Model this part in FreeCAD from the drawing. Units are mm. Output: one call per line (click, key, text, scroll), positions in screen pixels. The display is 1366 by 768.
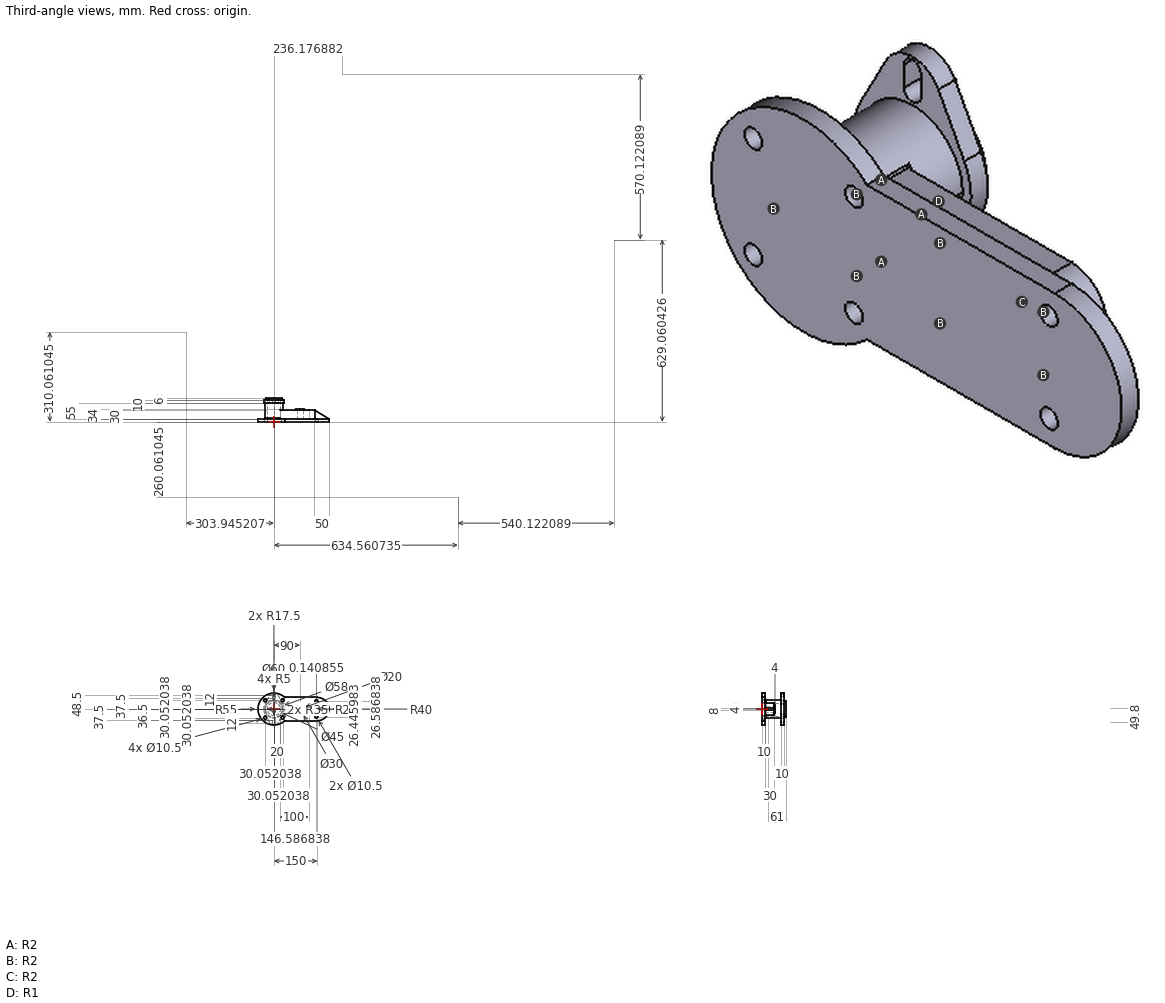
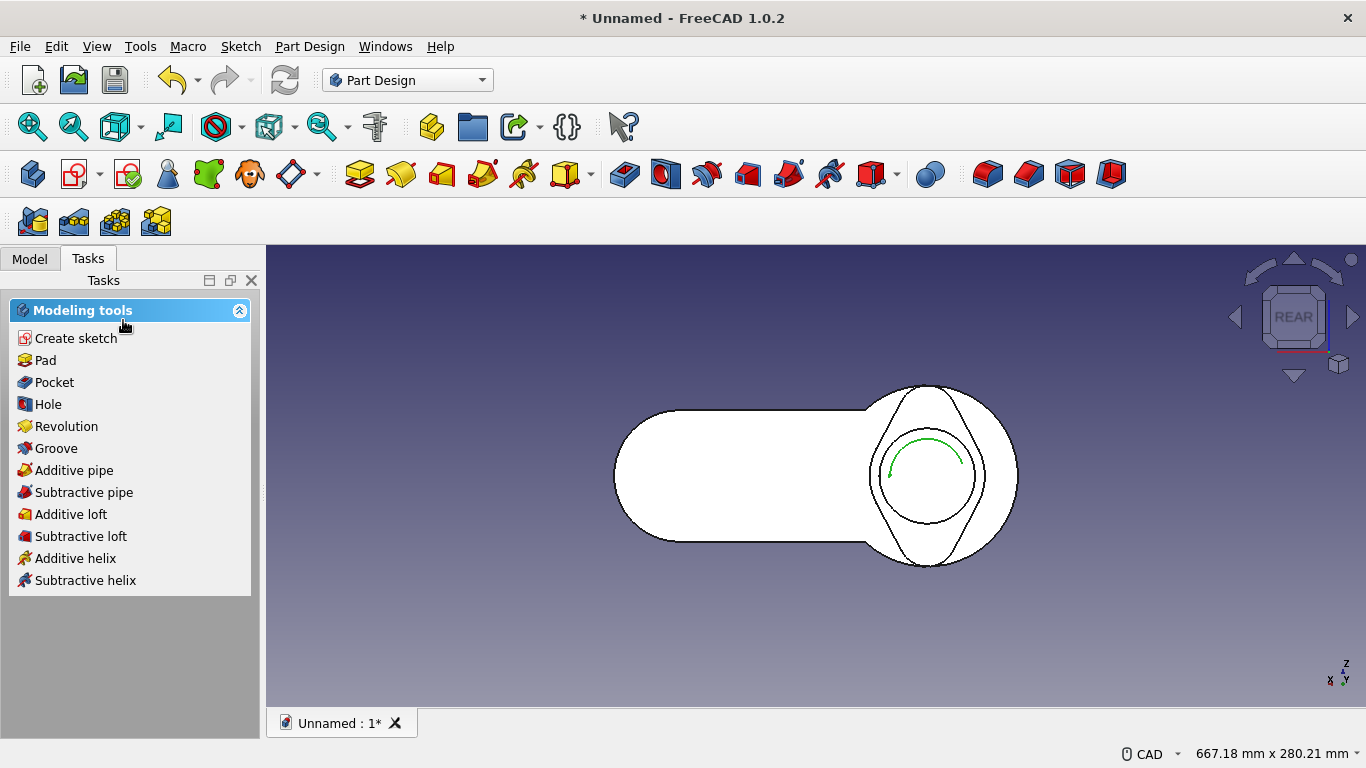
click(625, 174)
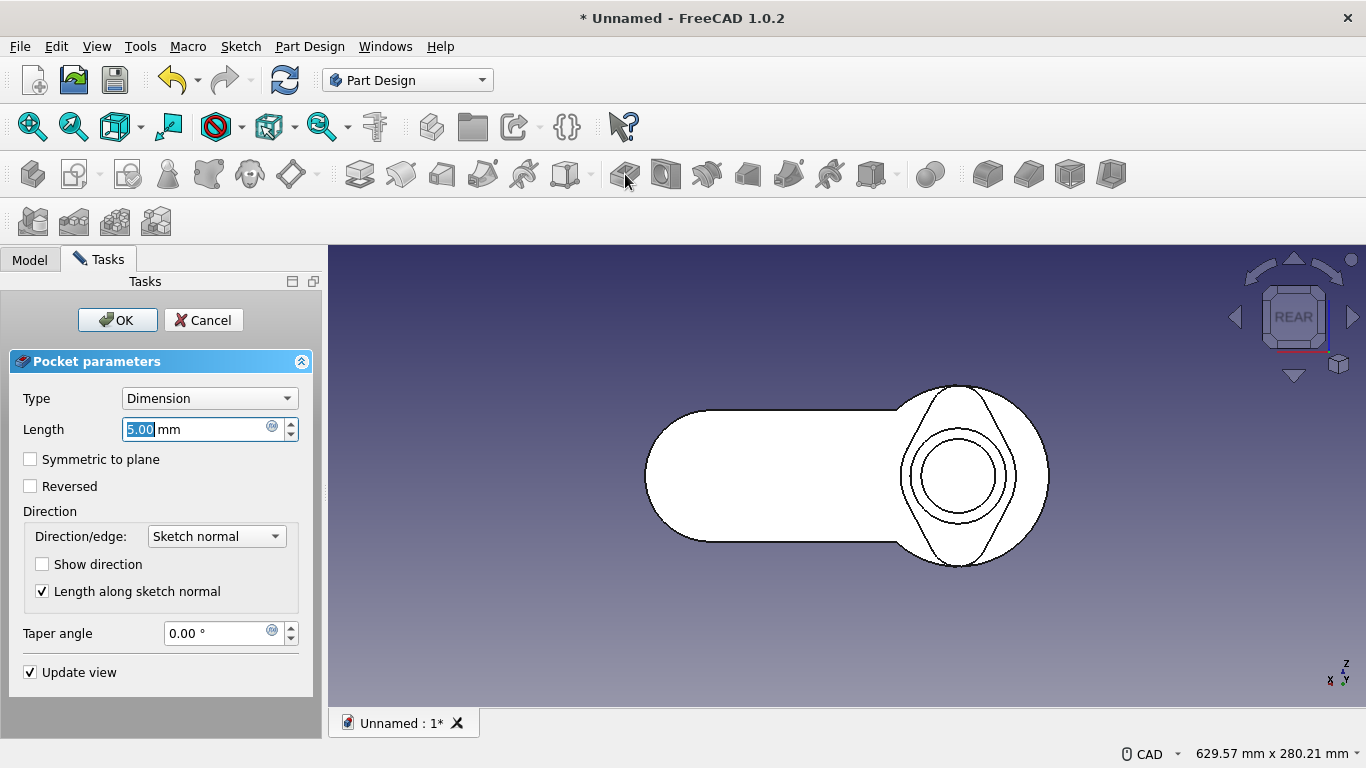
text(61)
key(Tab)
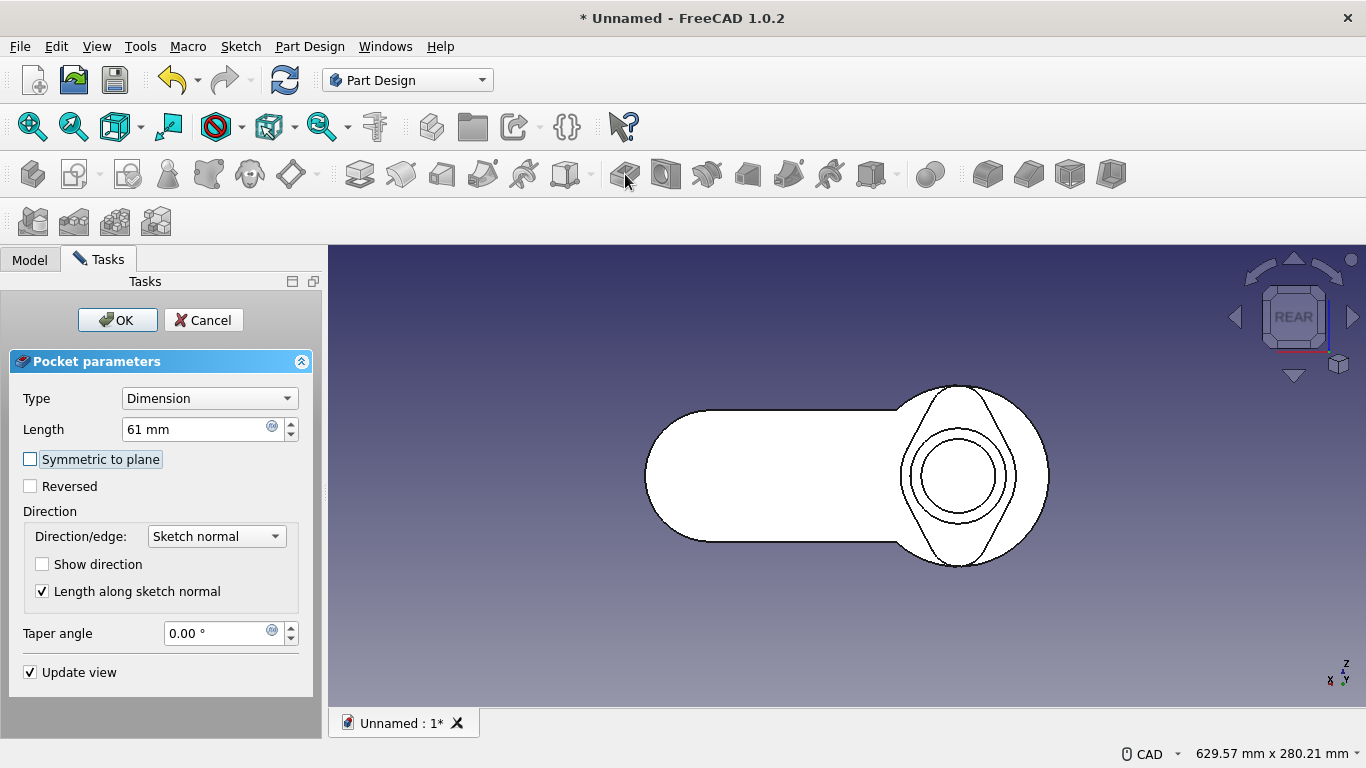
click(118, 320)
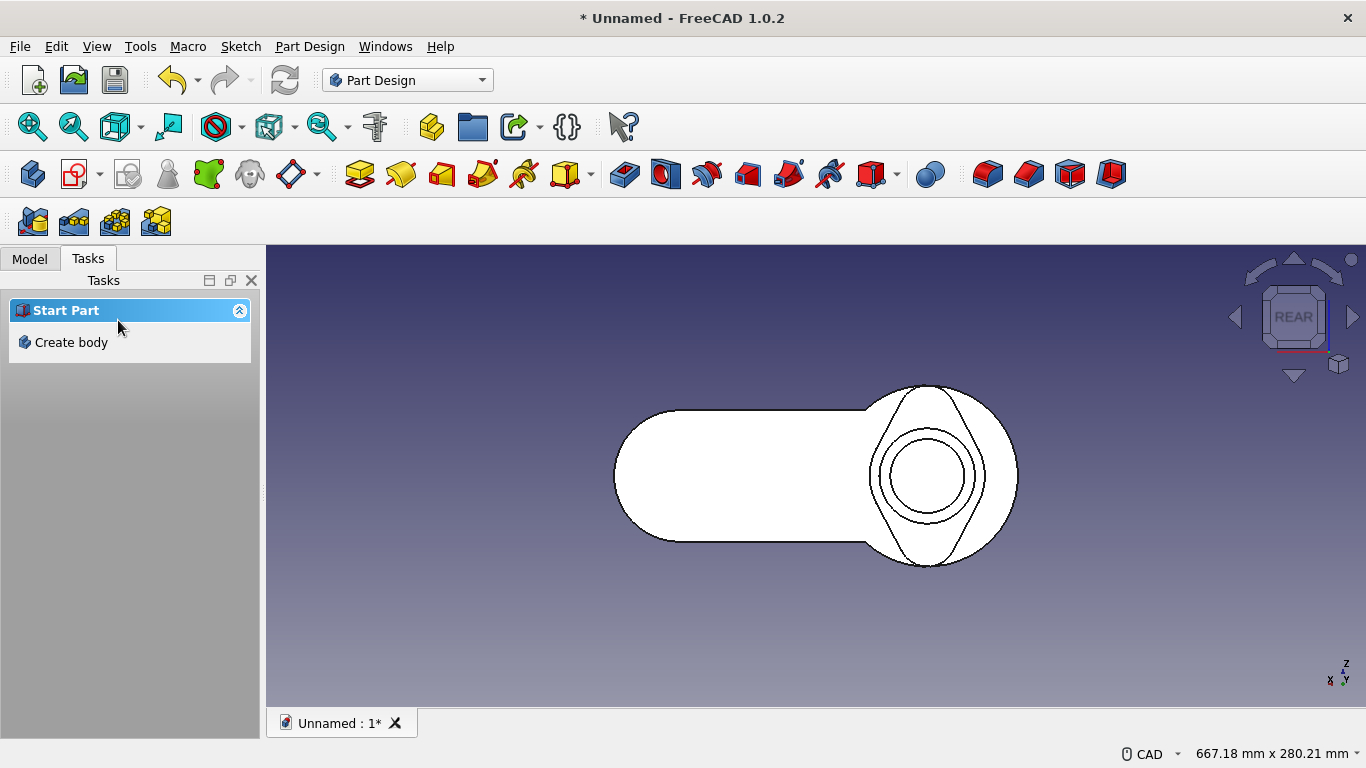
key(v)
key(f)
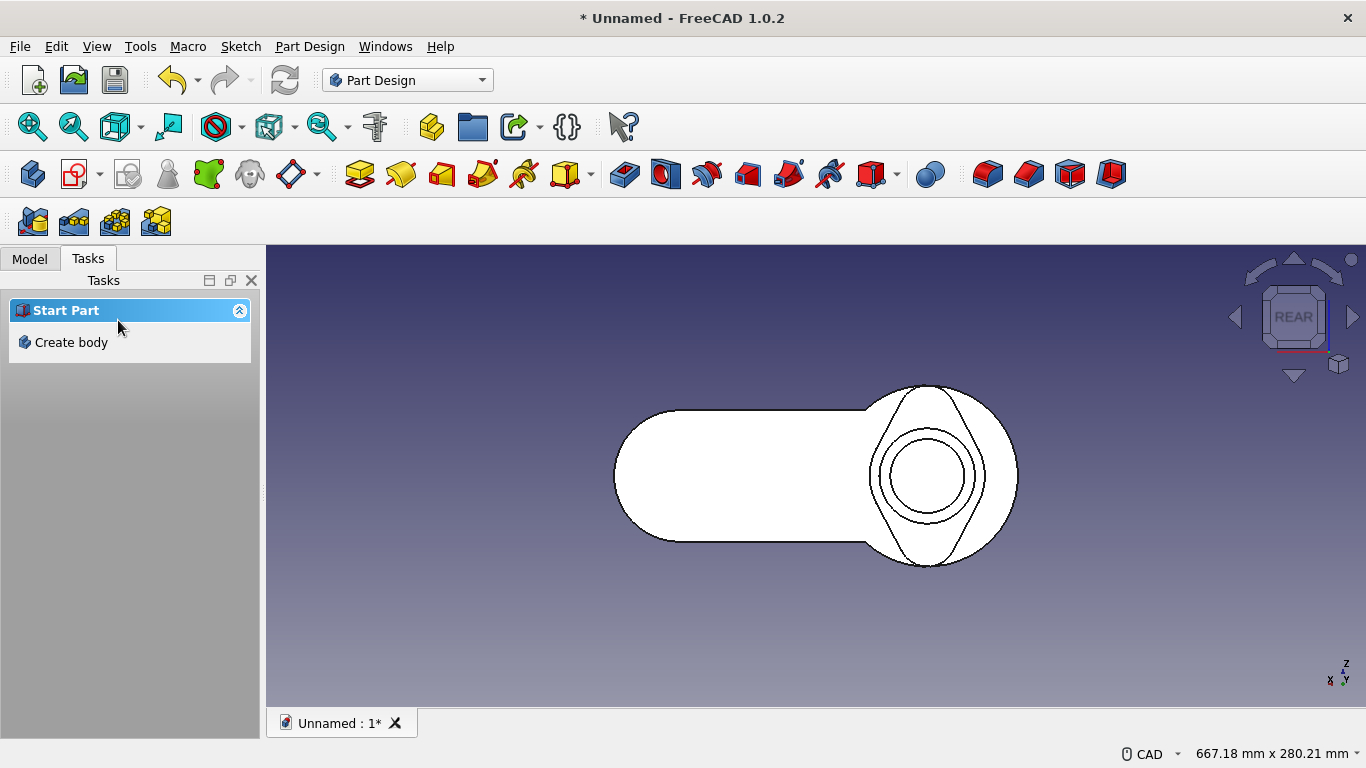
click(927, 397)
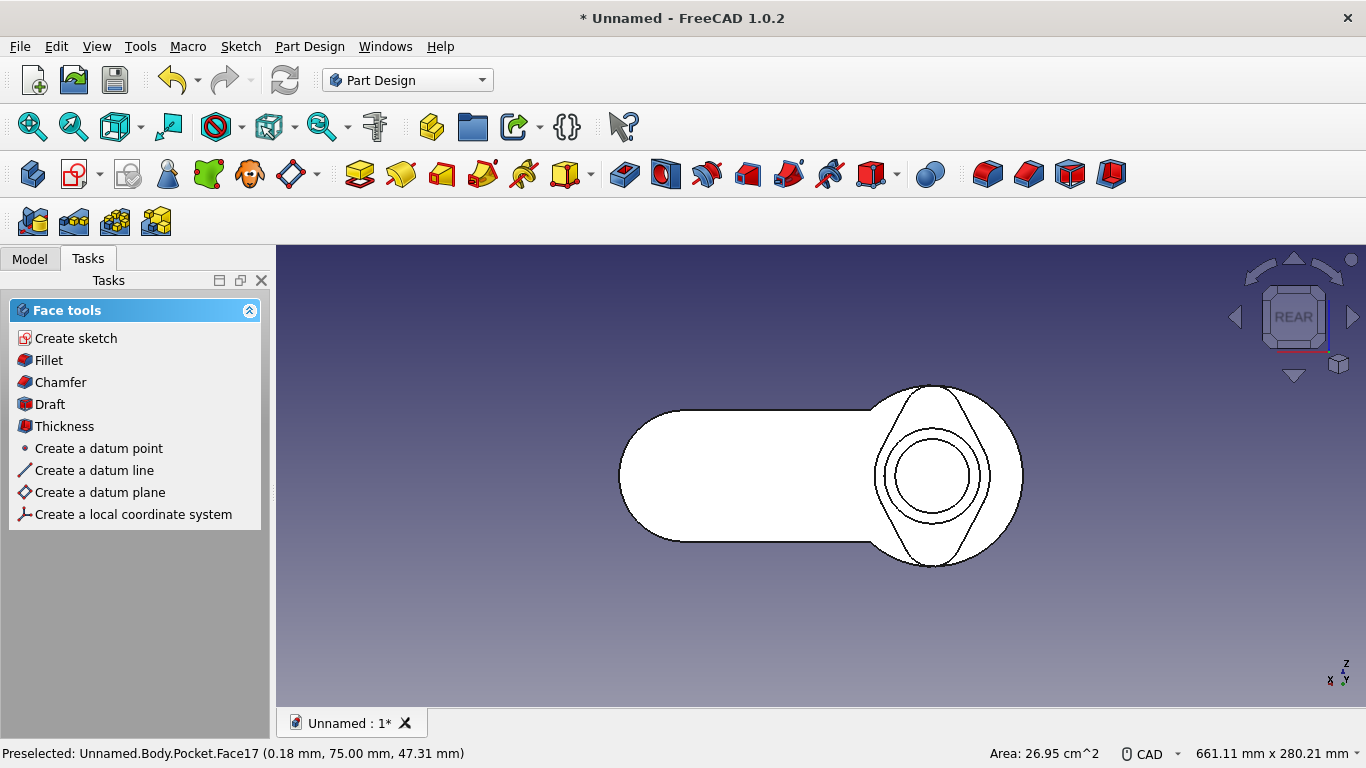
click(74, 174)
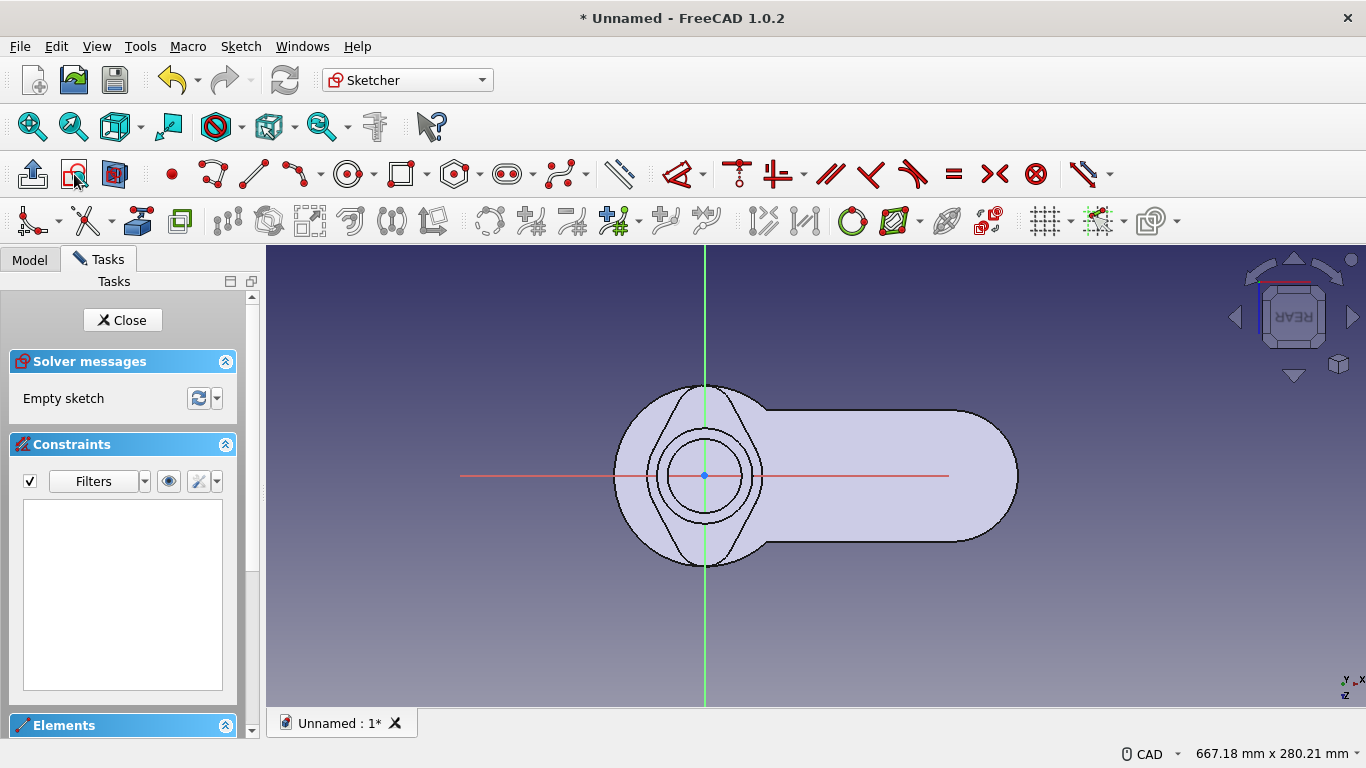
scroll(618, 476, up, 2)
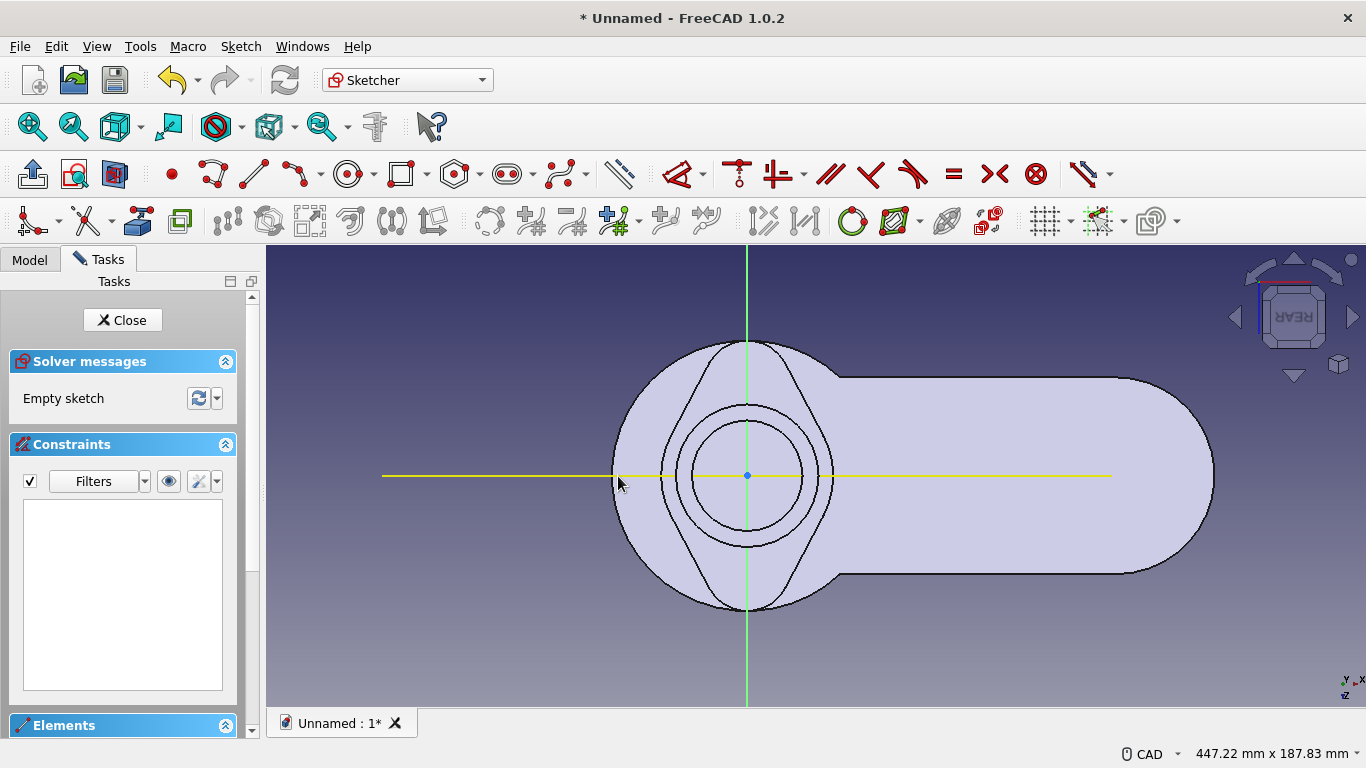
click(506, 174)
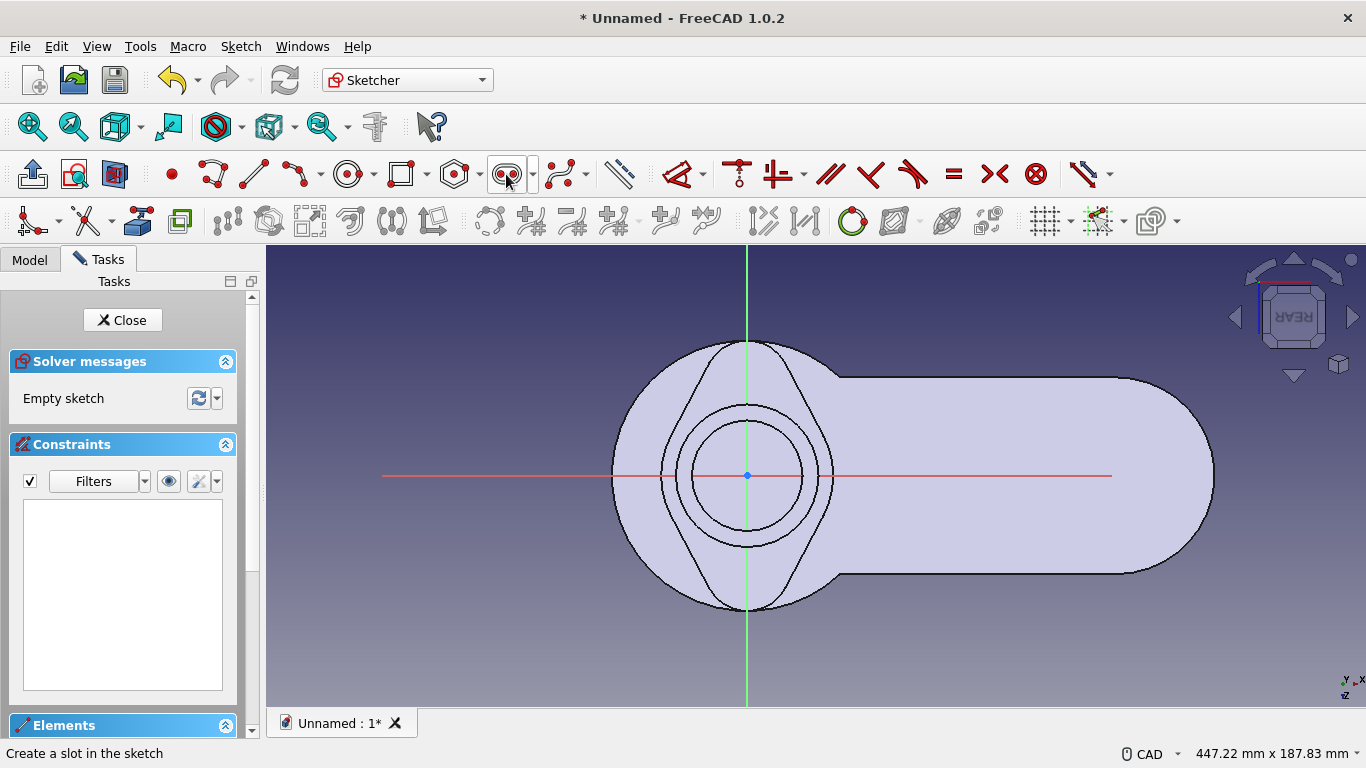
scroll(747, 386, up, 4)